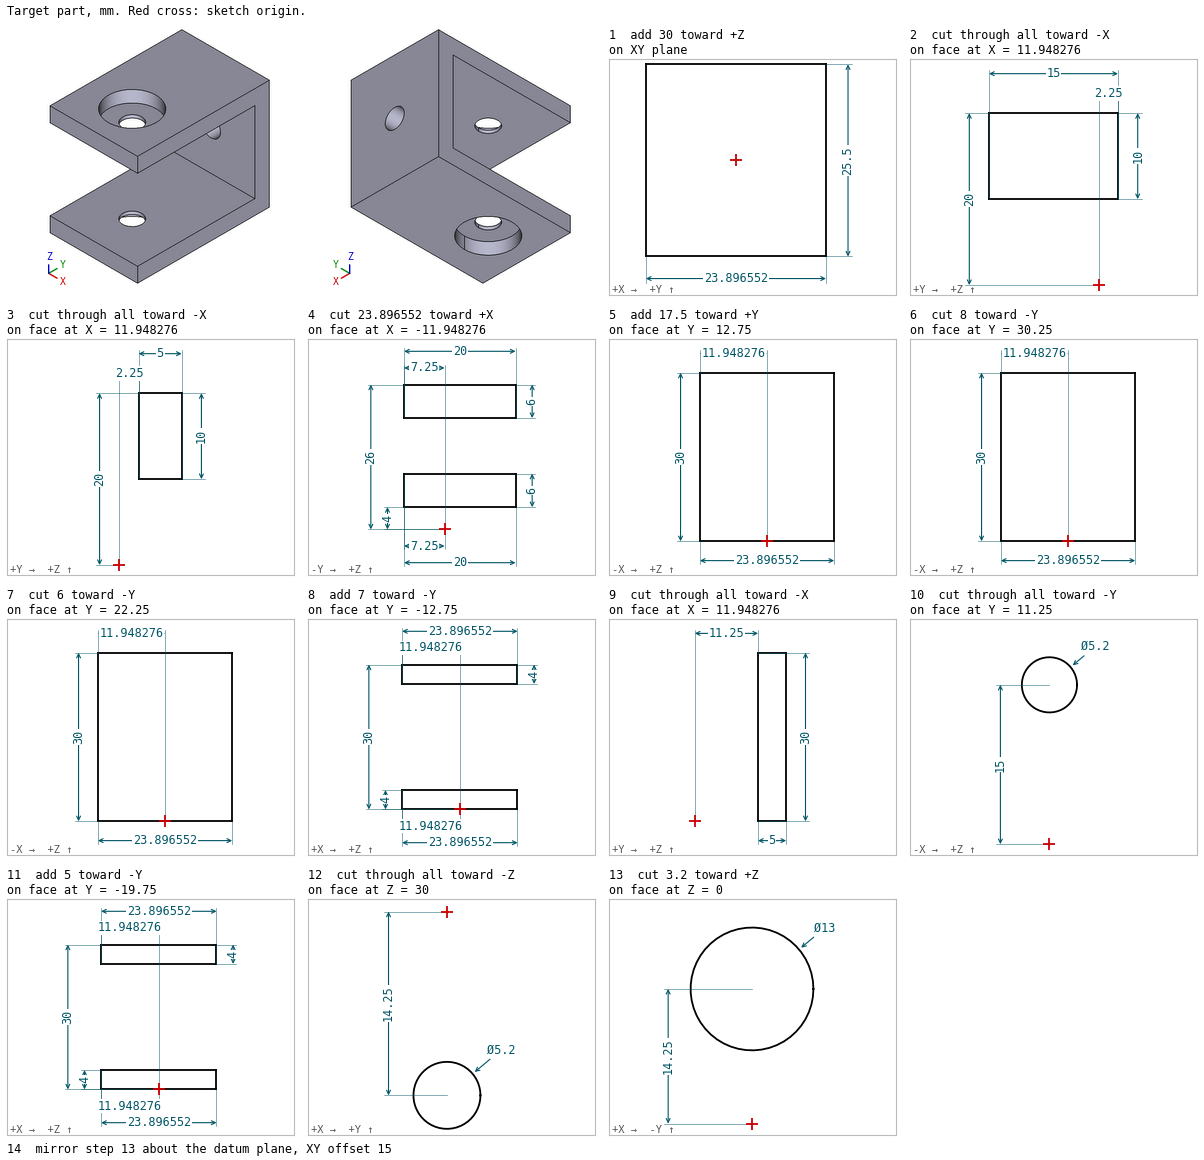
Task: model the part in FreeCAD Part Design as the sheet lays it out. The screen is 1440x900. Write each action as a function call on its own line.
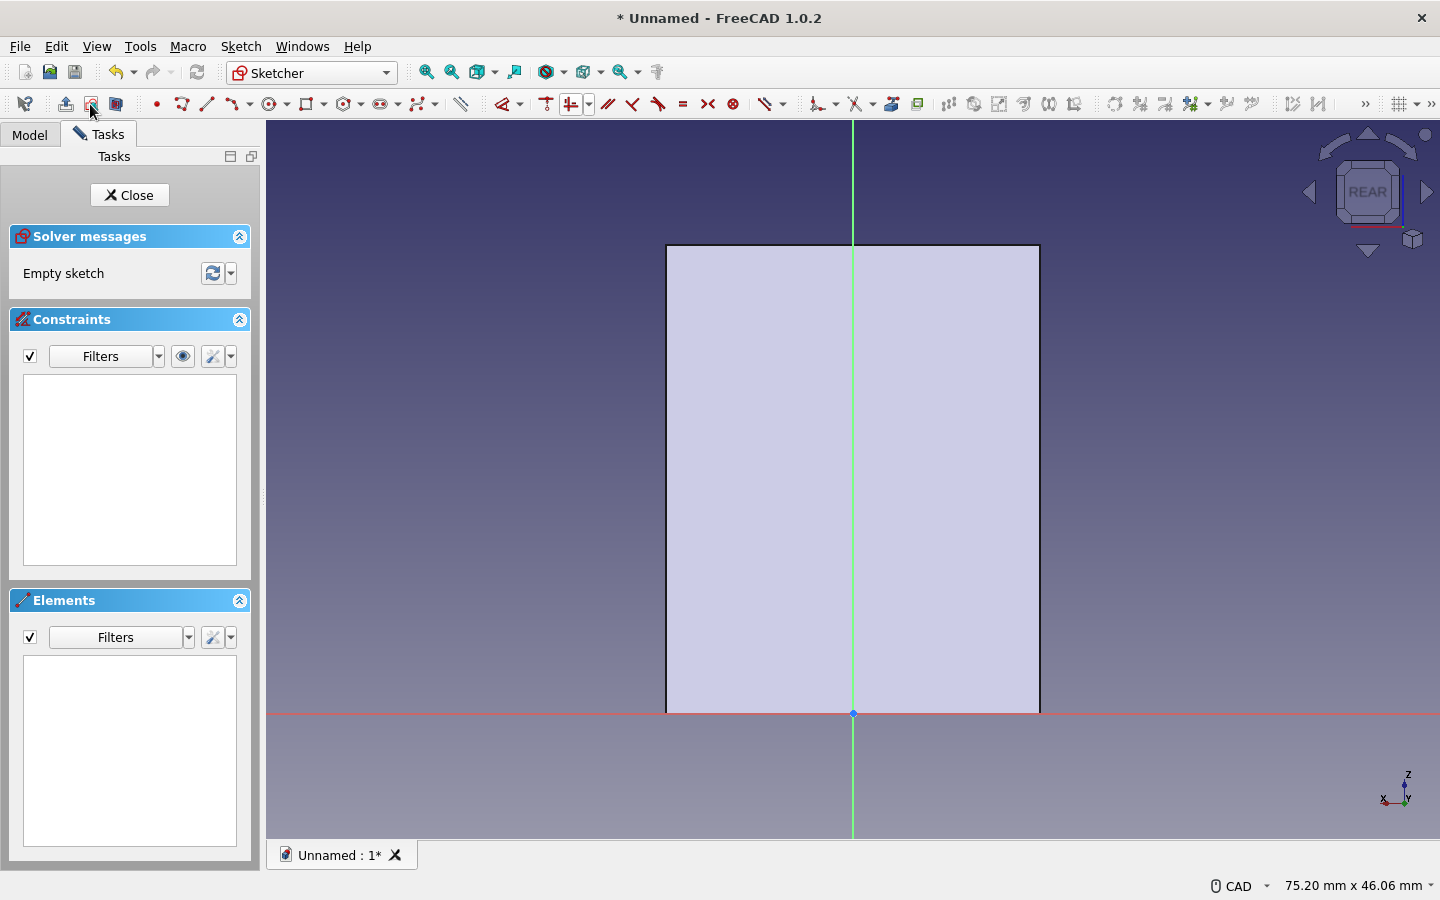
key(g)
key(r)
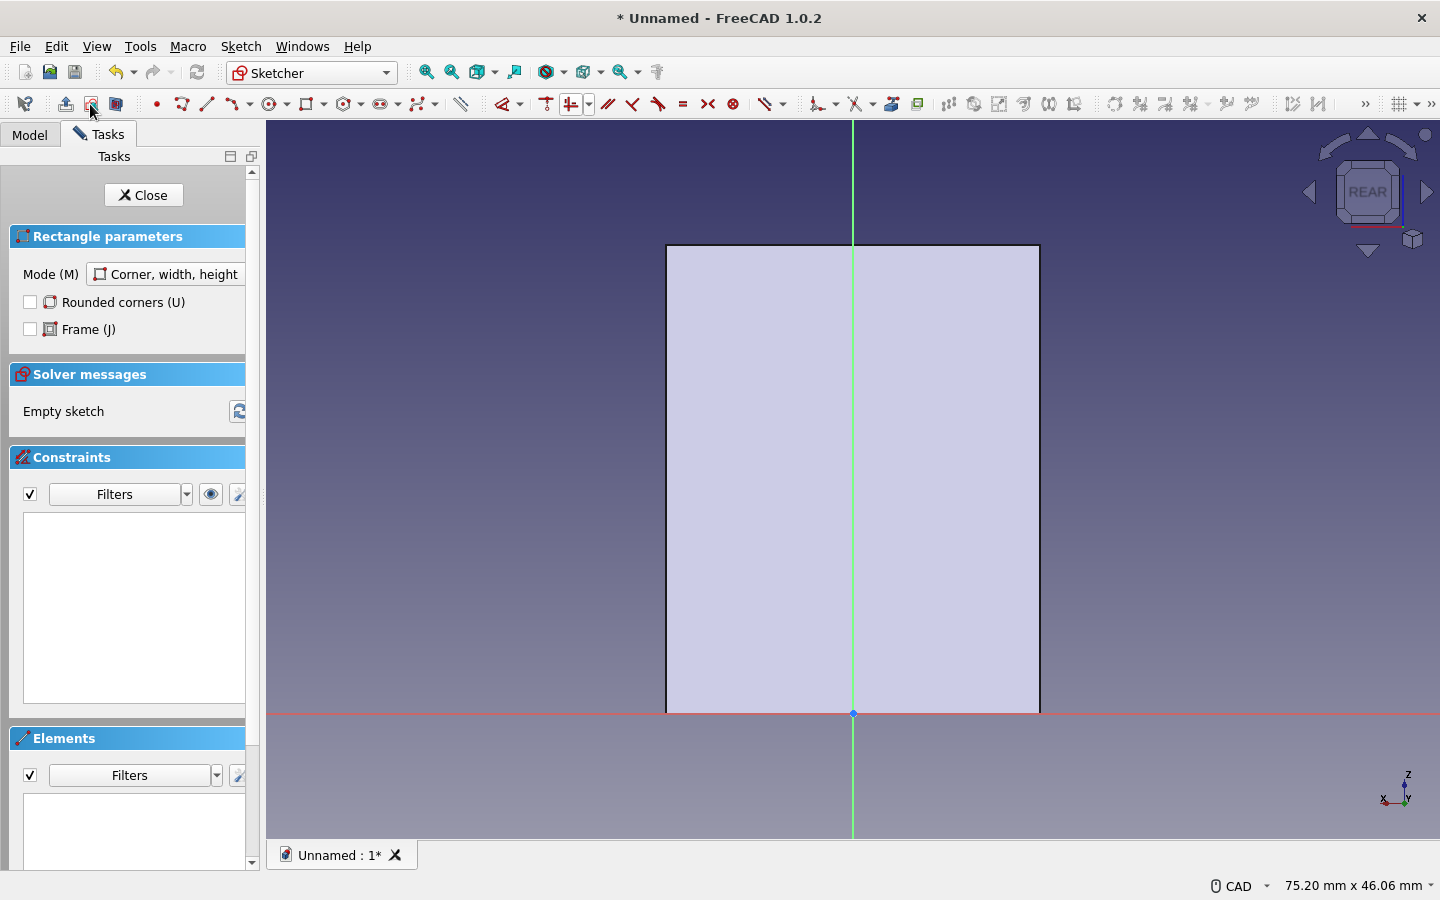
click(666, 245)
click(1040, 714)
key(Escape)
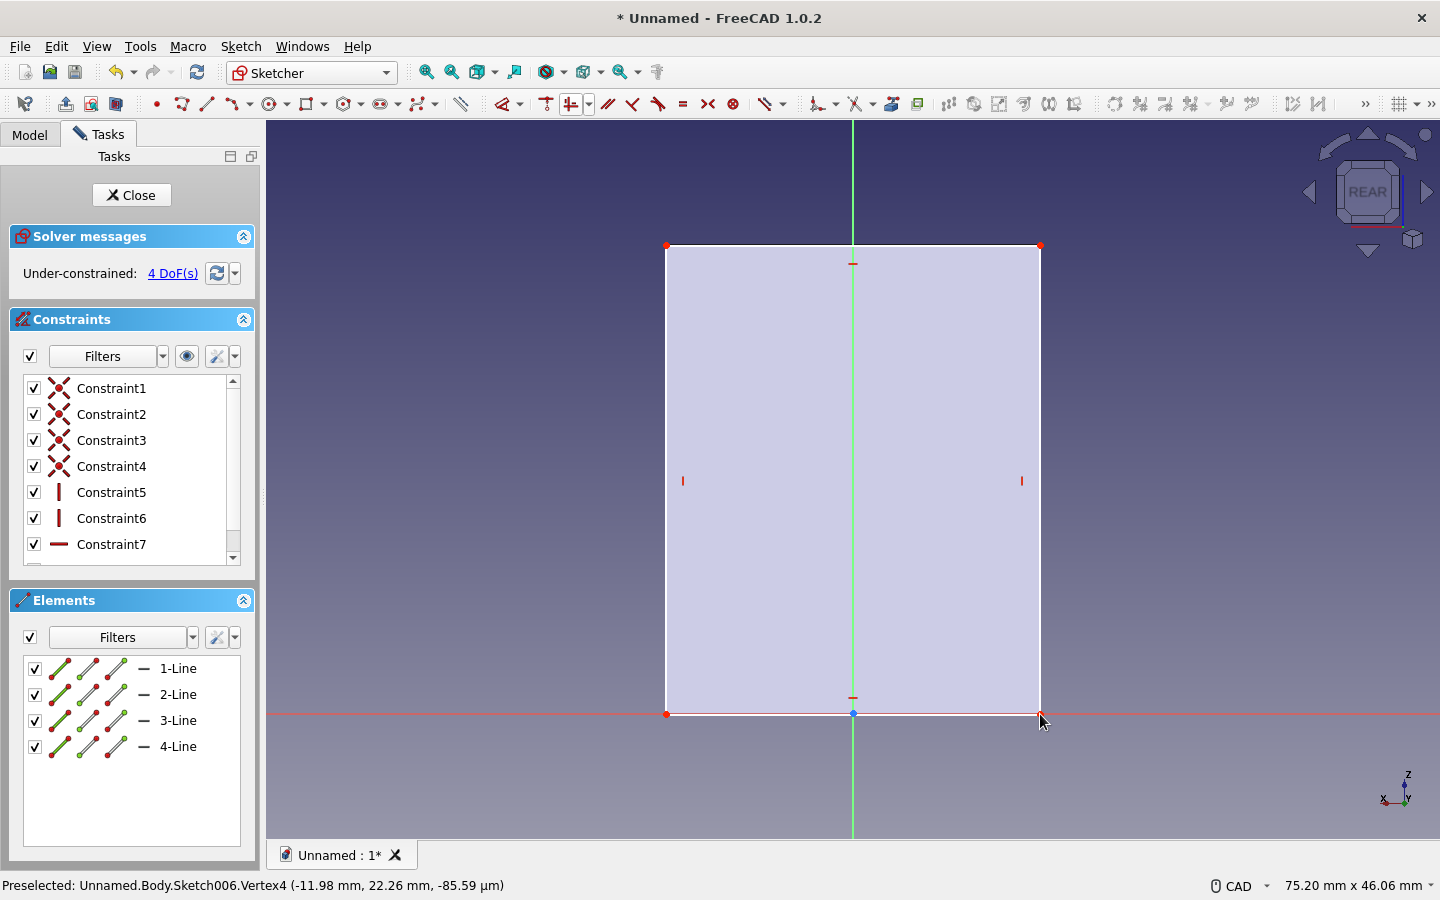
click(666, 715)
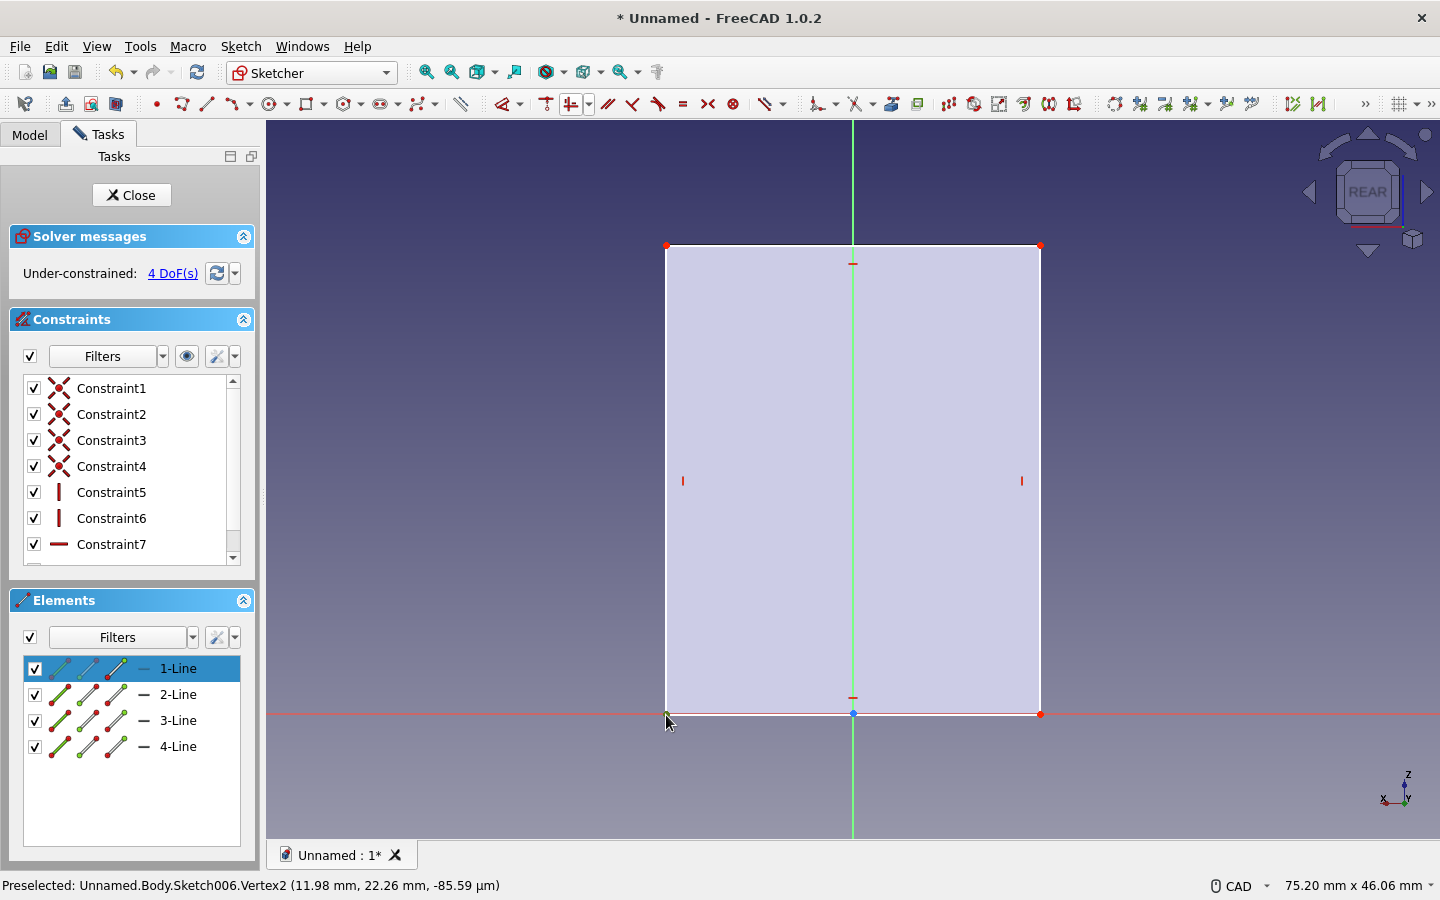
click(364, 714)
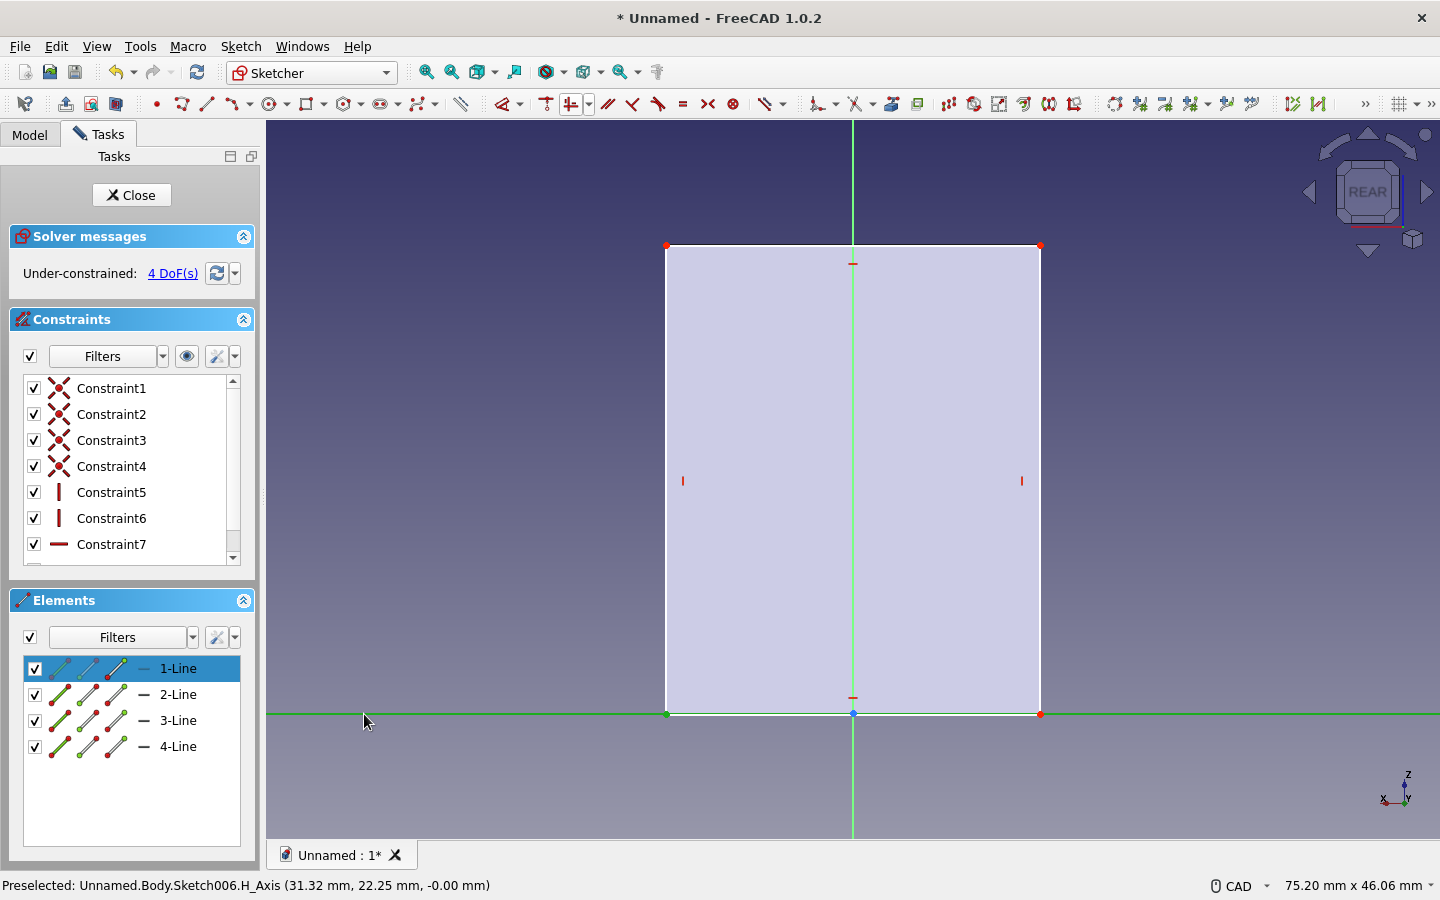
key(c)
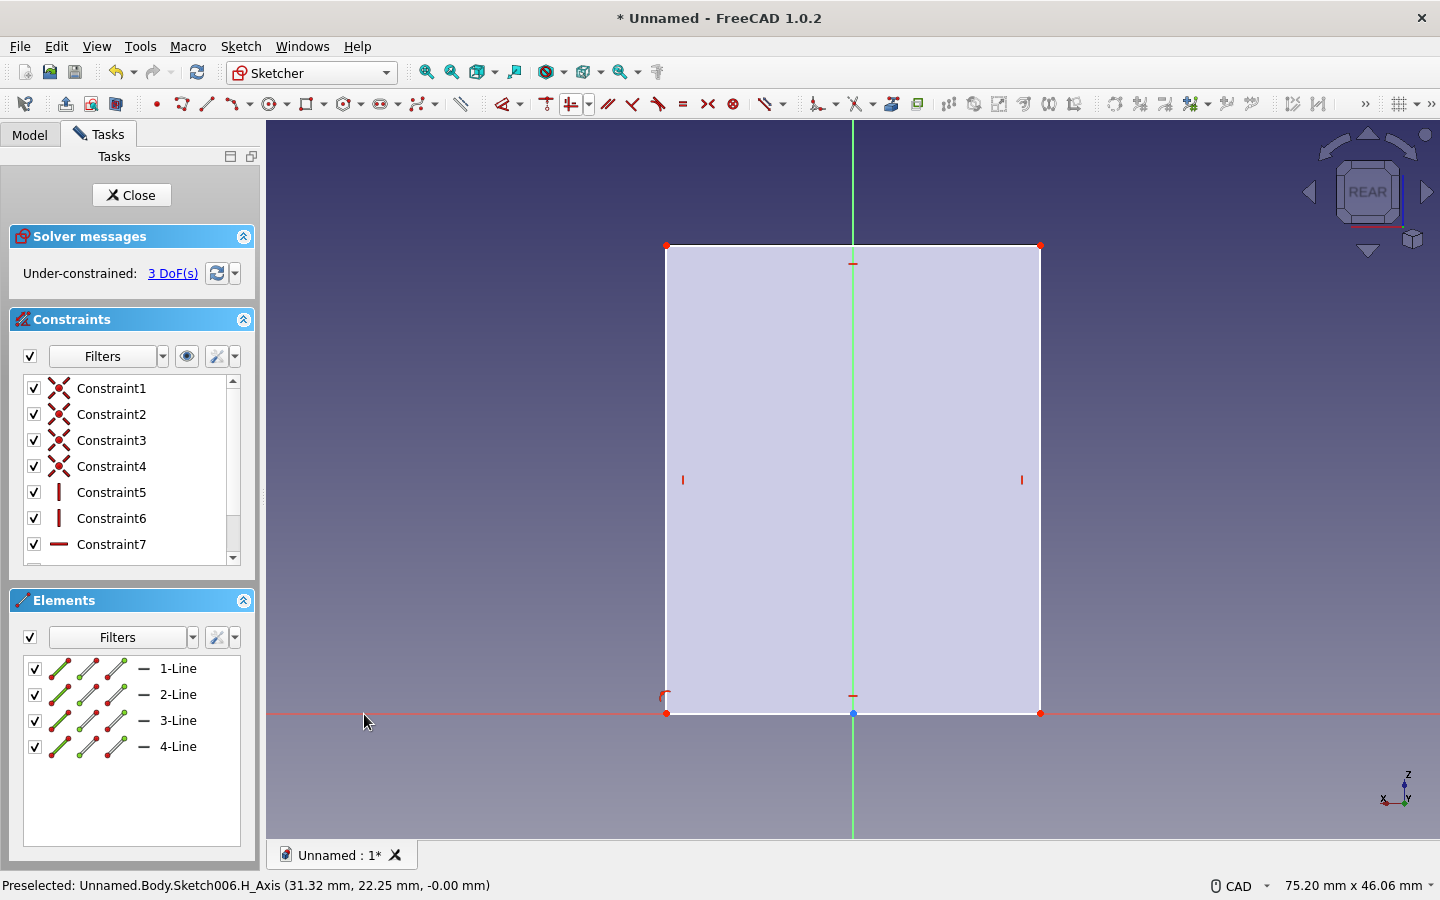
key(d)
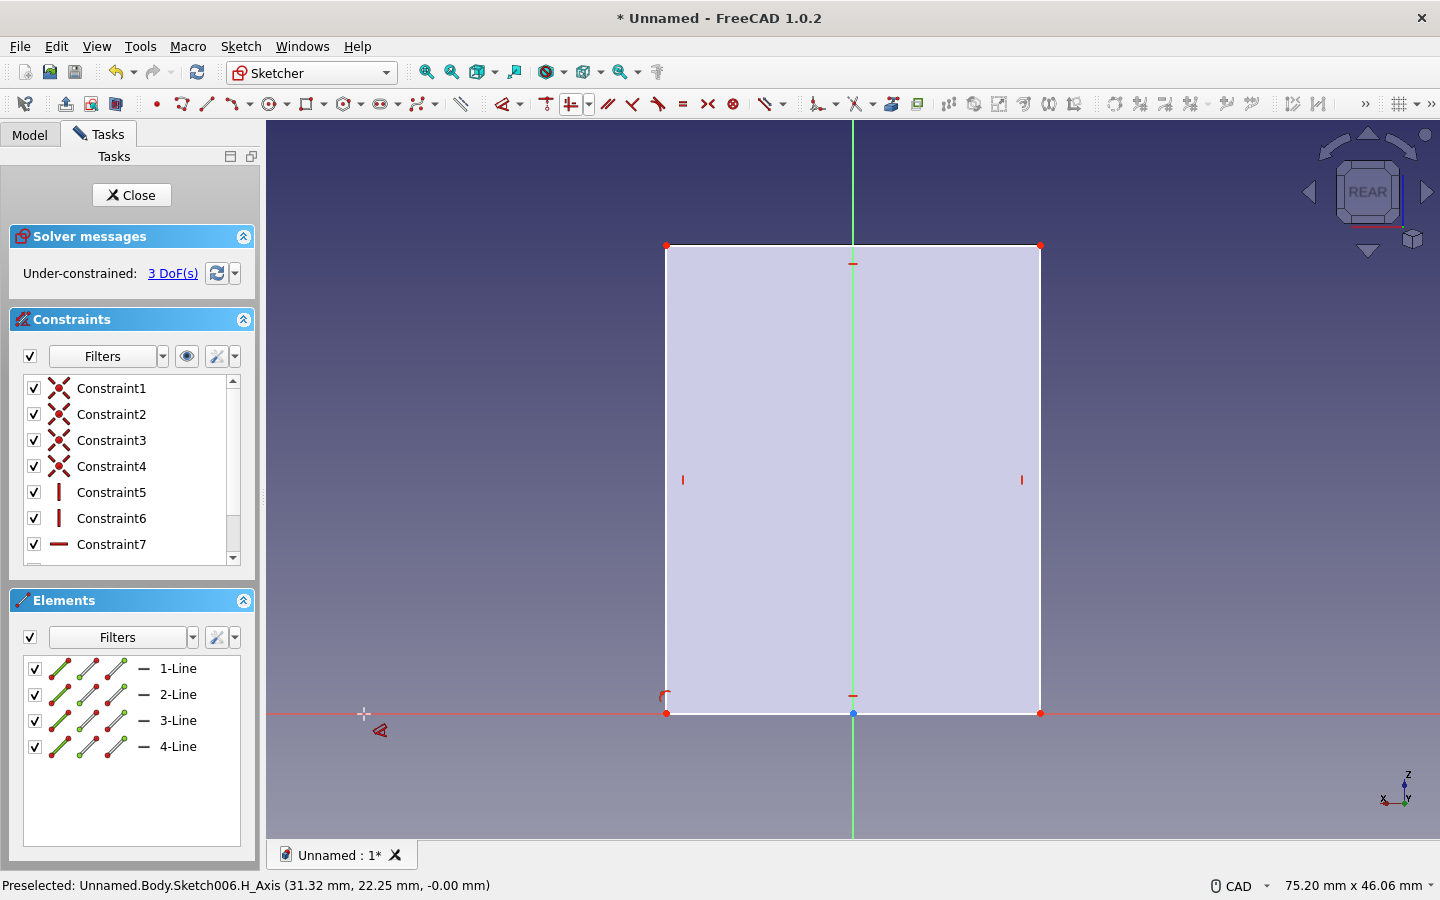
click(666, 386)
click(632, 480)